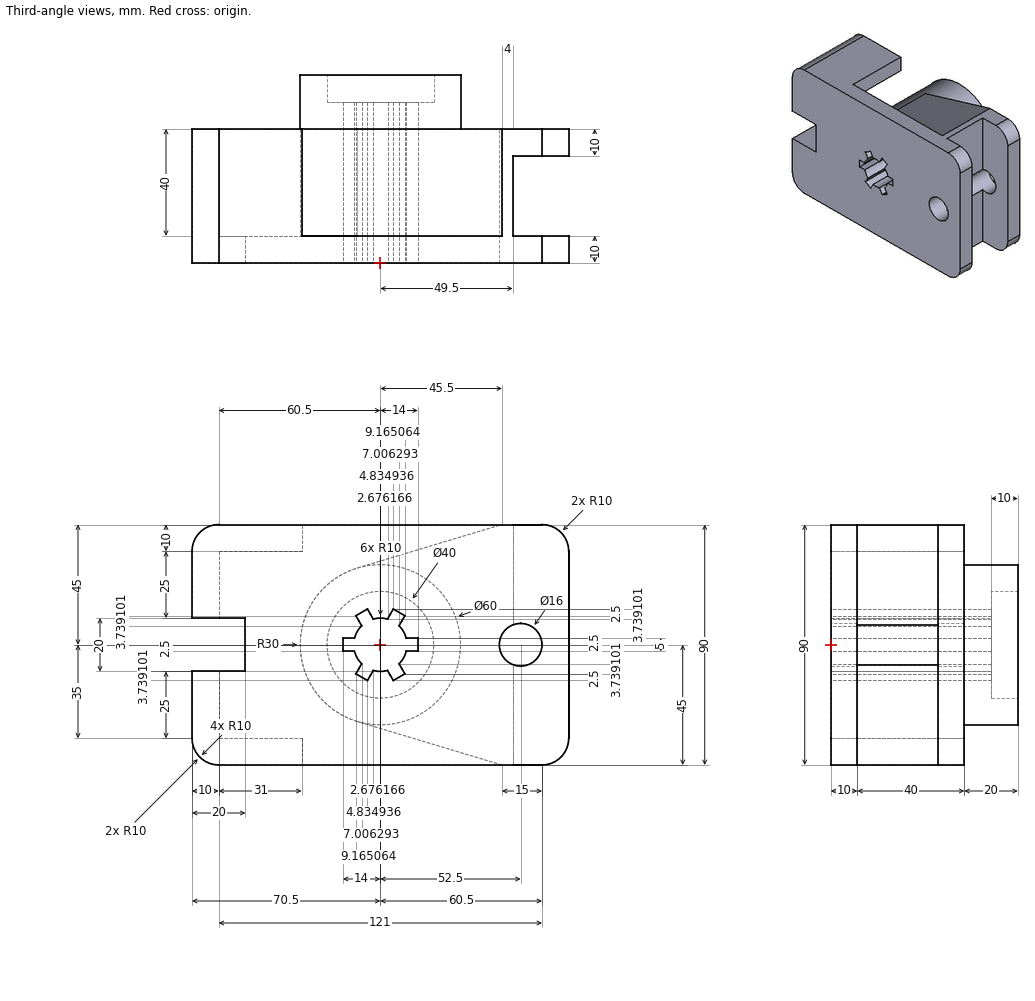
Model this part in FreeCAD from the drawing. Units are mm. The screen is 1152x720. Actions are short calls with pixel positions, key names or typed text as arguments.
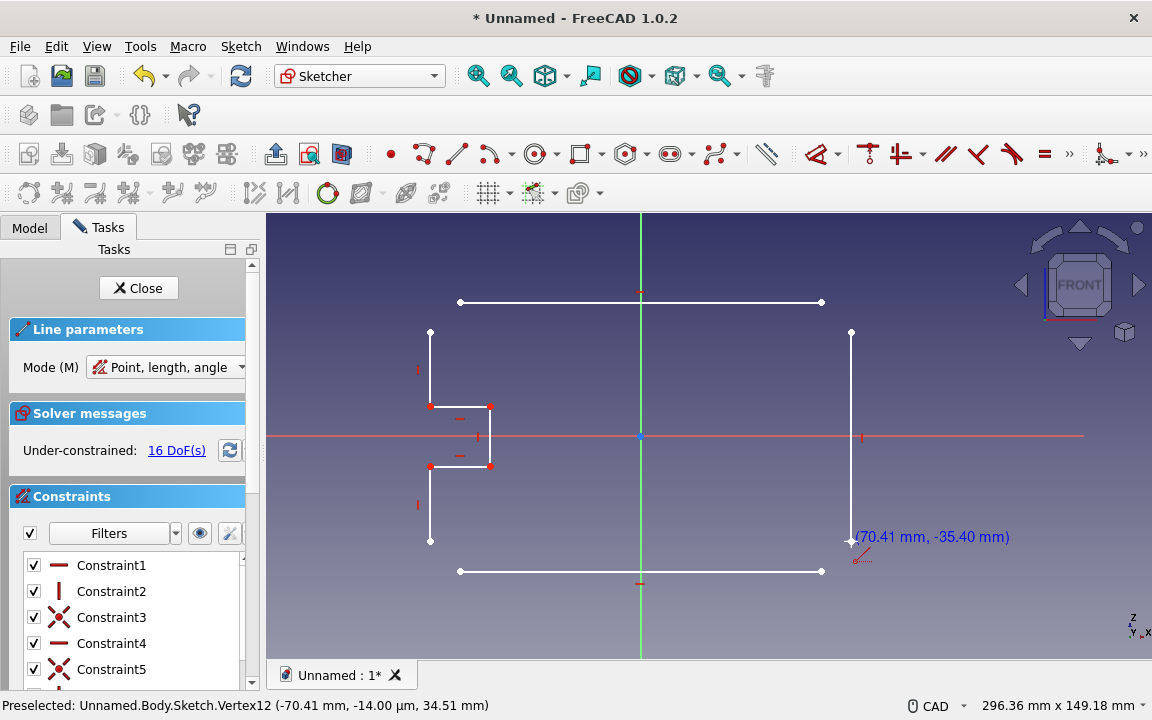
click(512, 154)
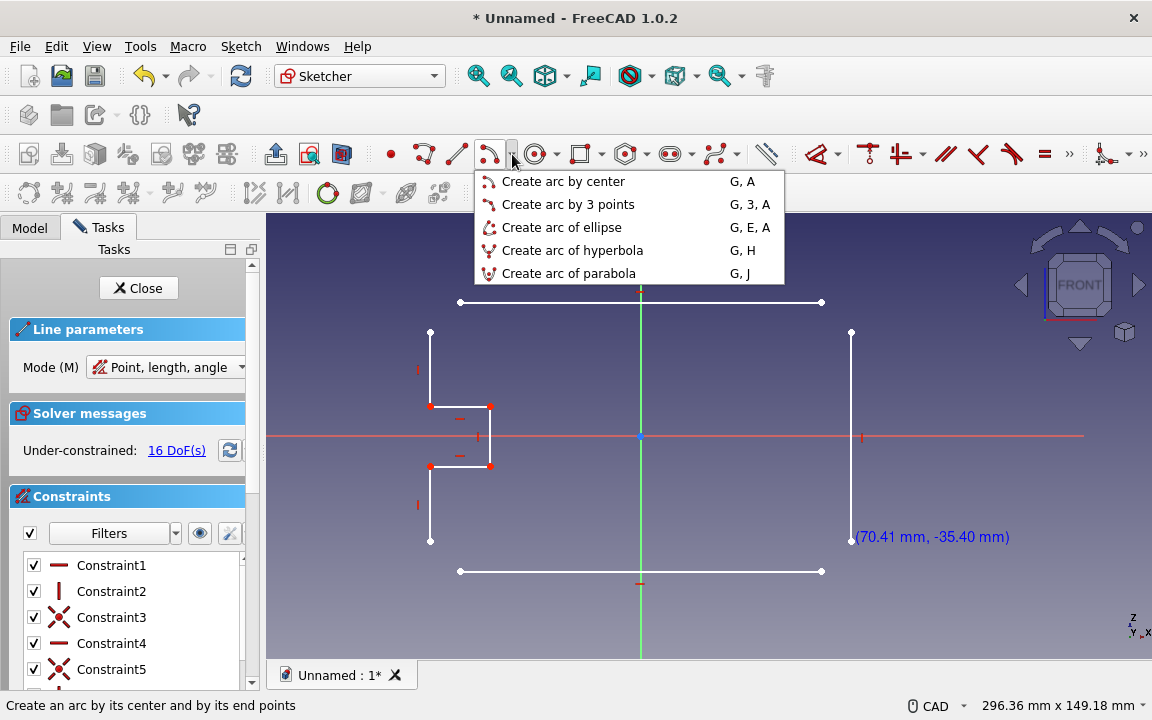
click(630, 204)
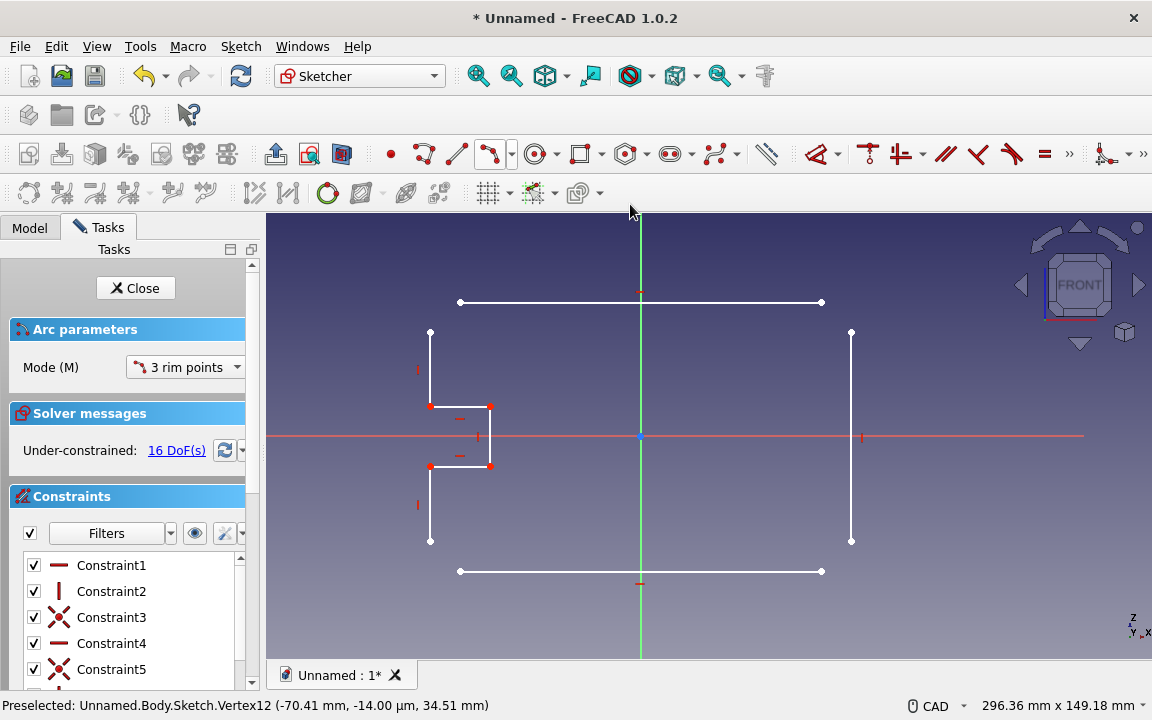
click(460, 572)
click(430, 542)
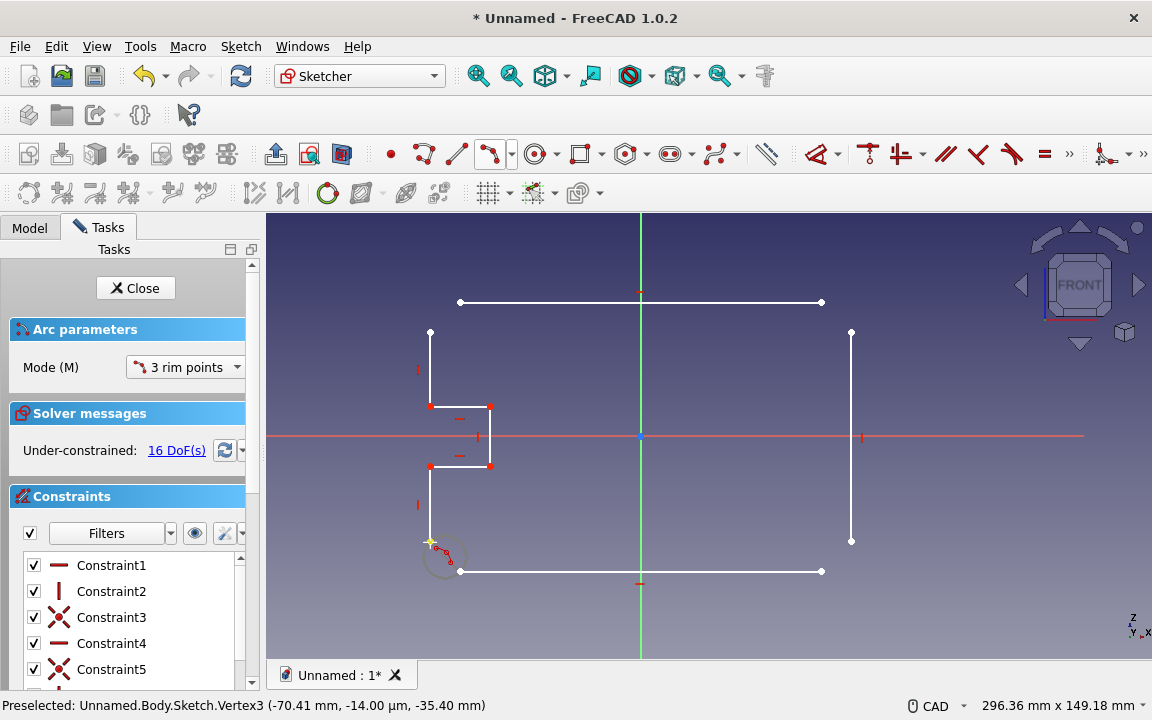
scroll(439, 562, up, 3)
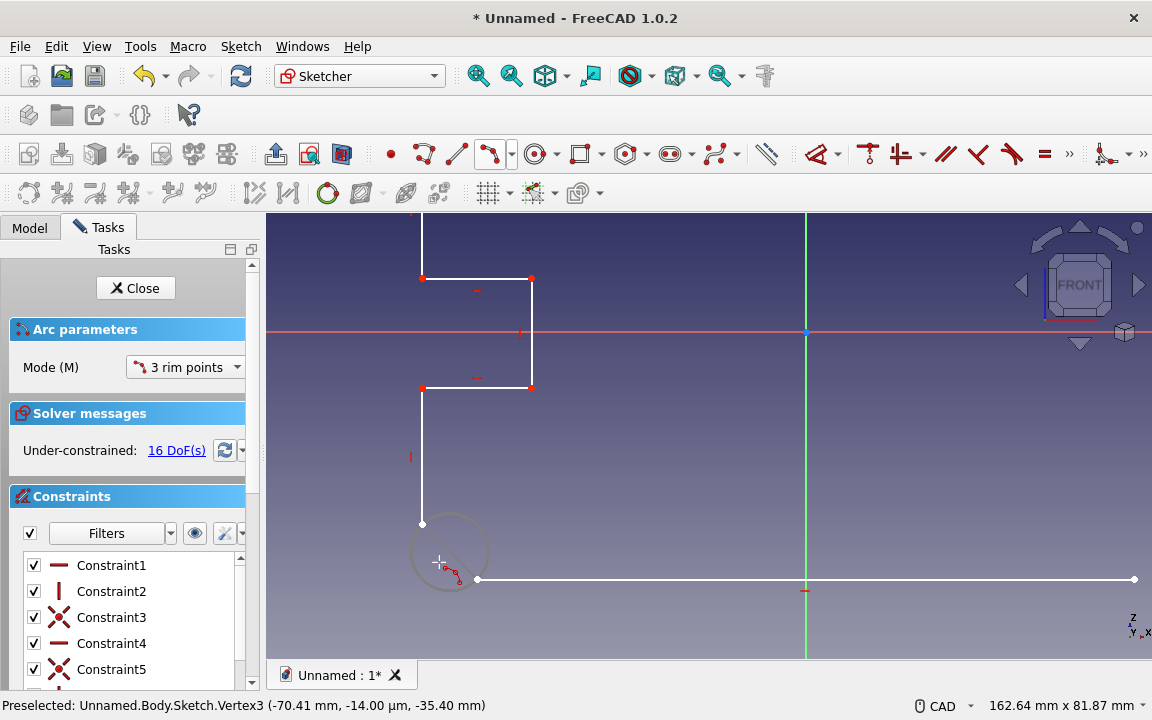
click(438, 561)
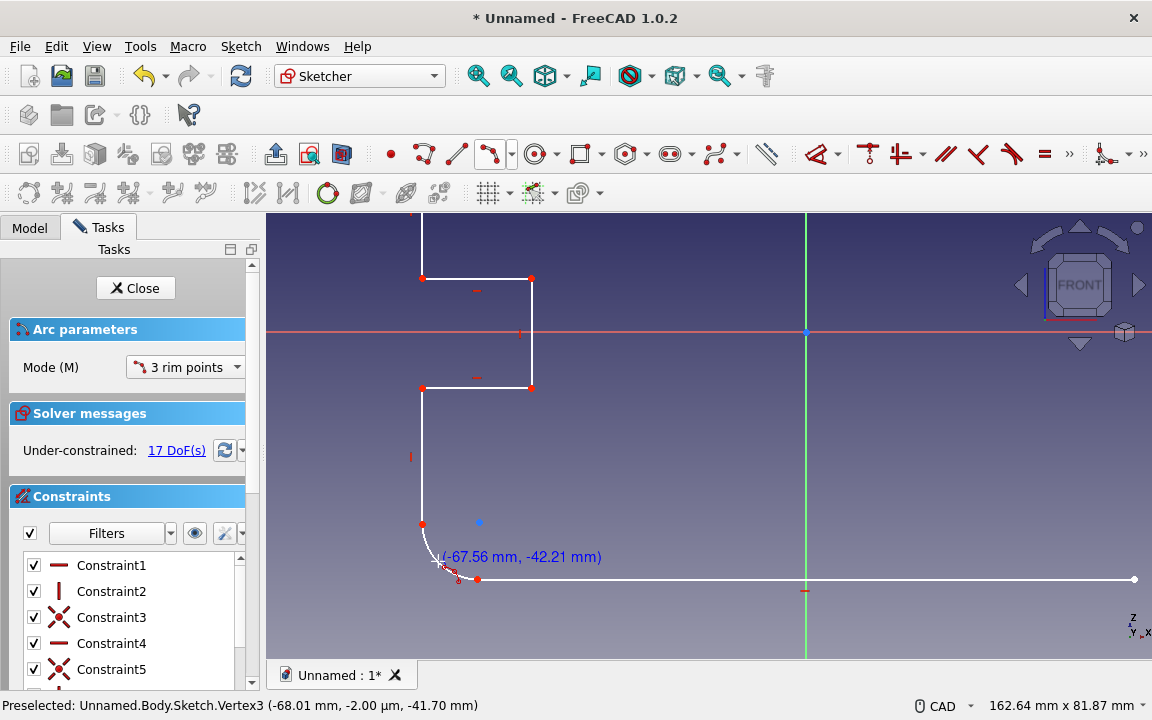
scroll(439, 562, down, 3)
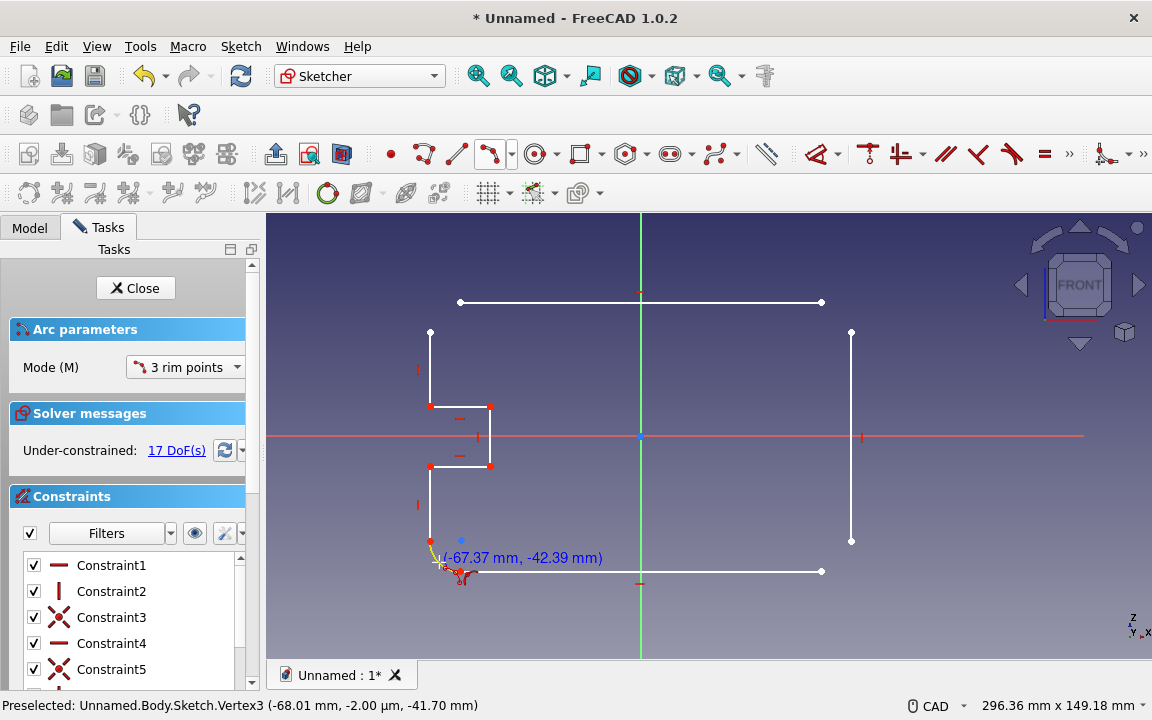
click(430, 333)
click(460, 303)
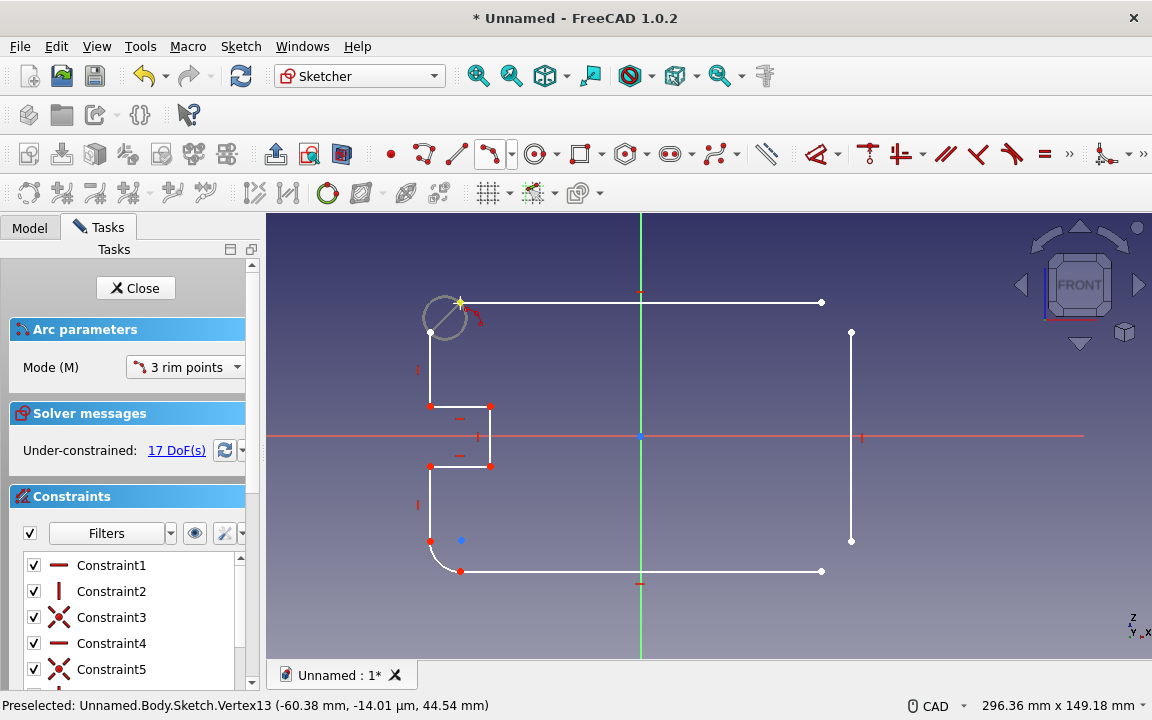
scroll(439, 310, up, 3)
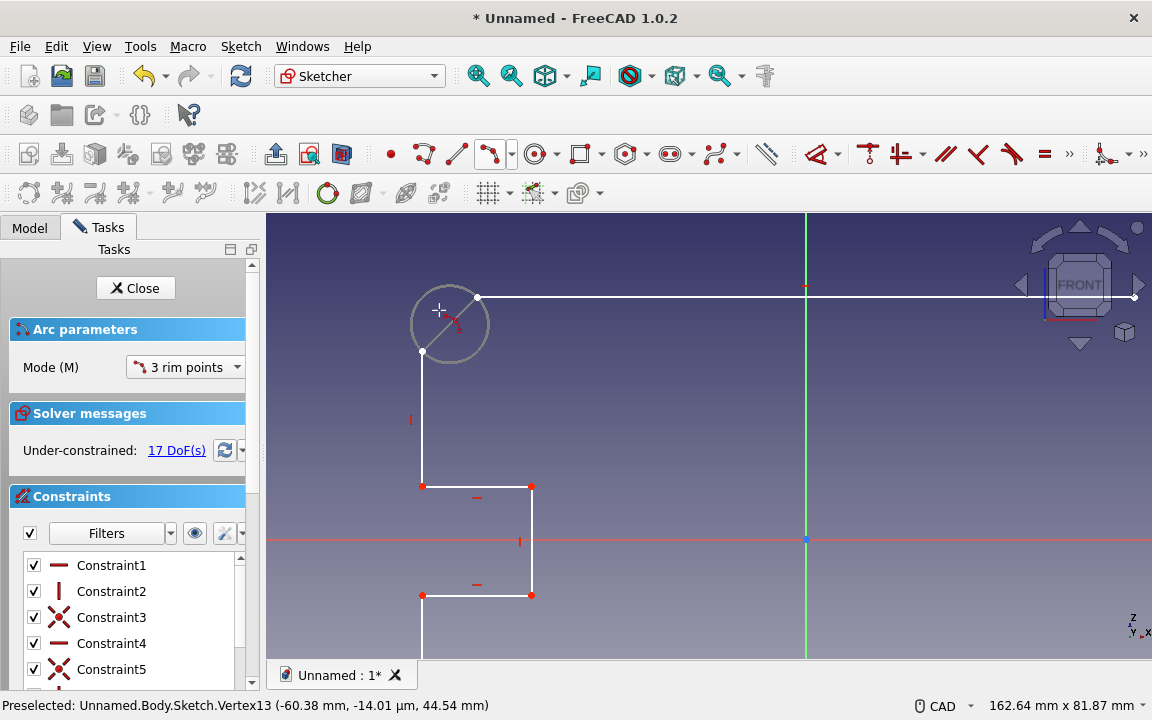
click(438, 311)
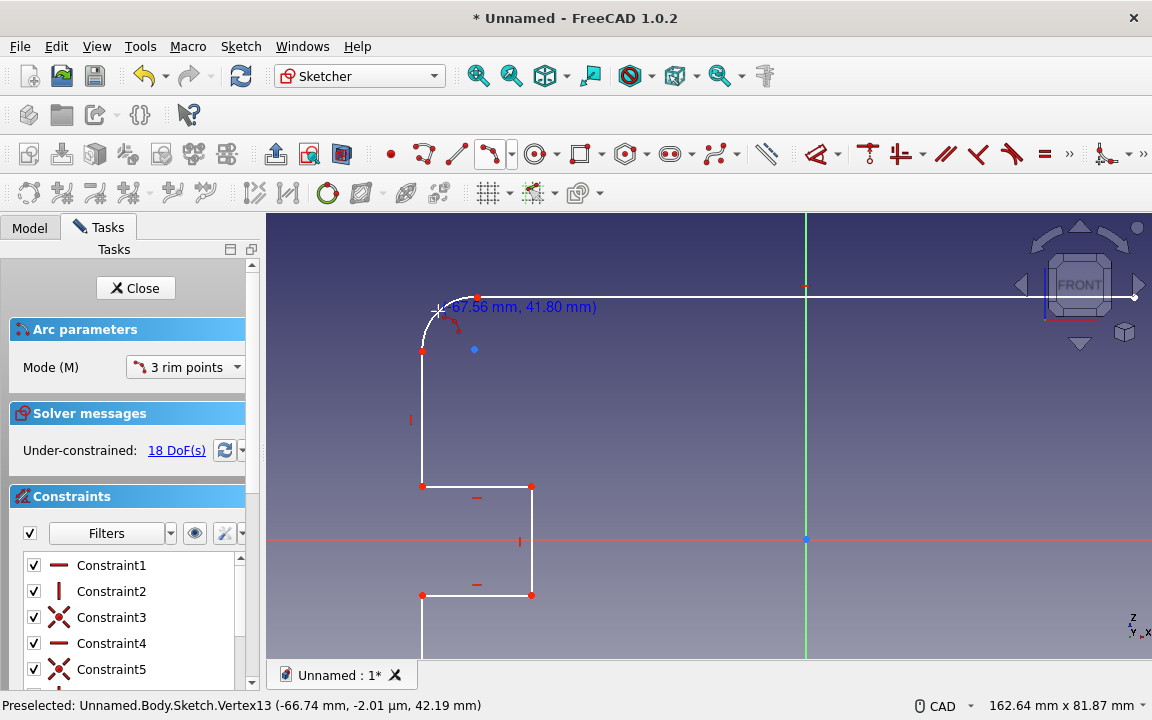
scroll(439, 310, down, 3)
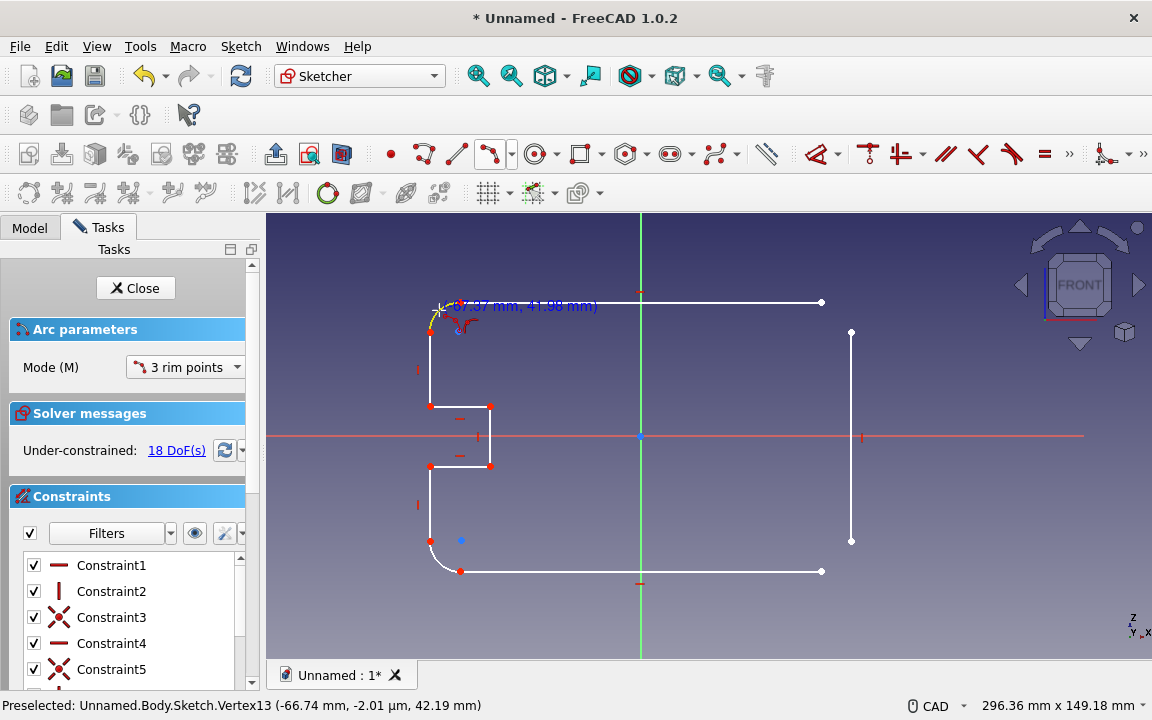
click(821, 303)
click(851, 333)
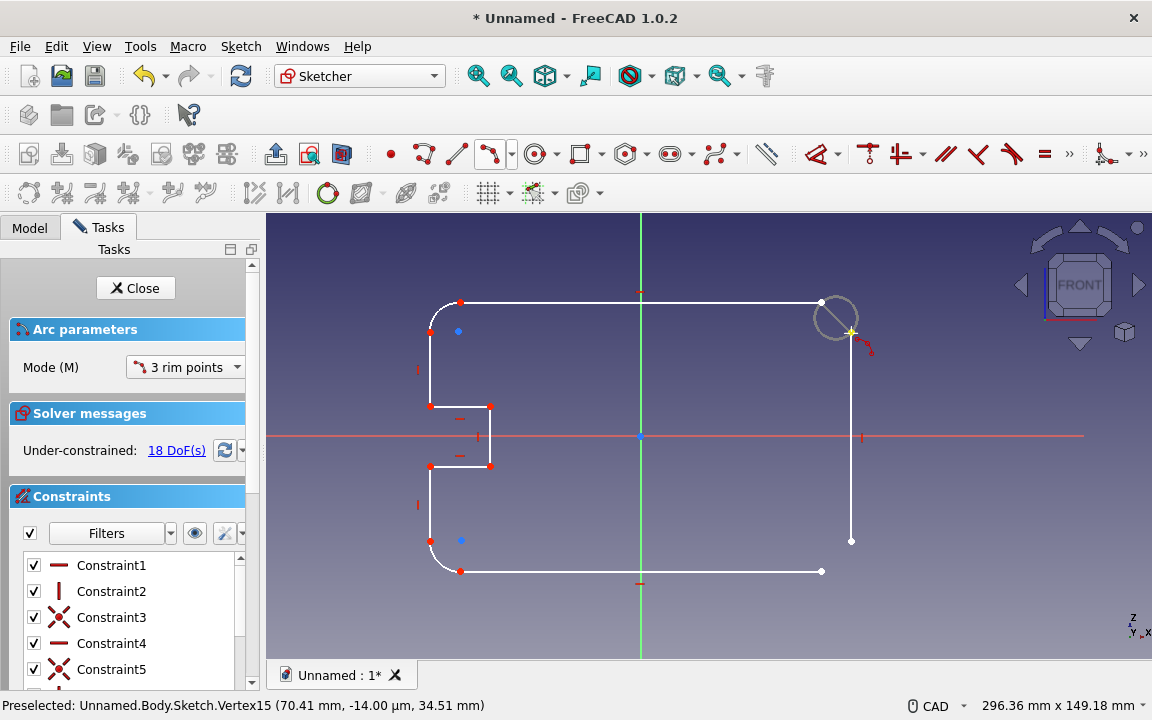
scroll(843, 310, up, 3)